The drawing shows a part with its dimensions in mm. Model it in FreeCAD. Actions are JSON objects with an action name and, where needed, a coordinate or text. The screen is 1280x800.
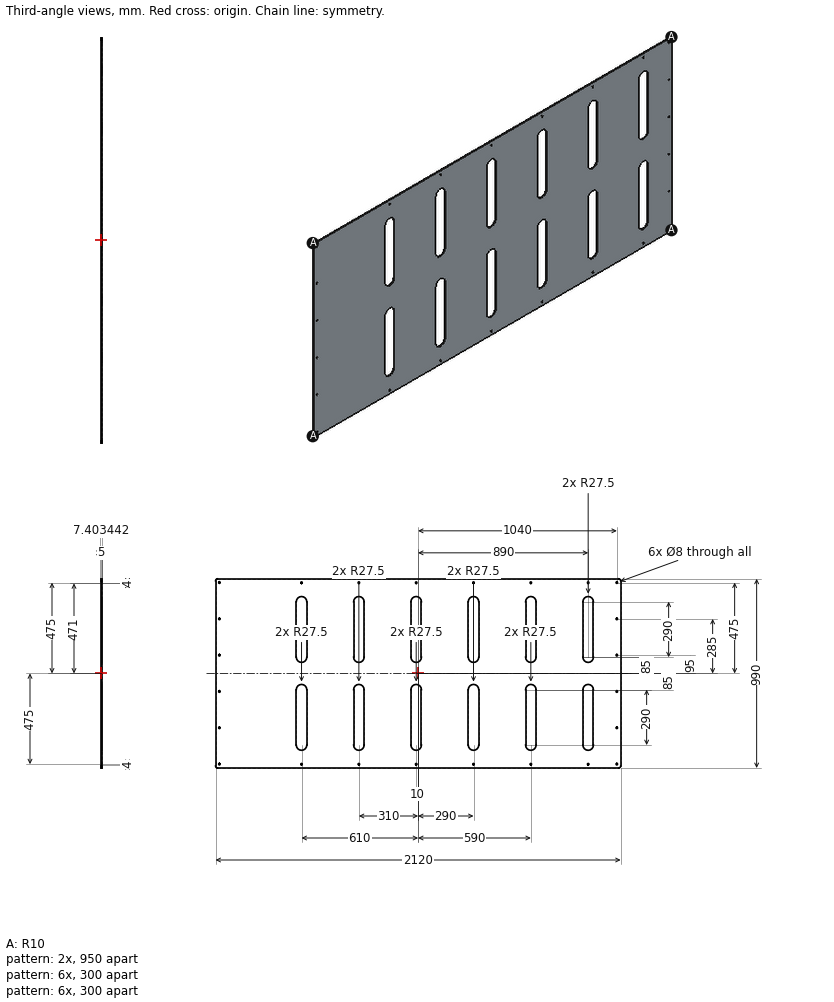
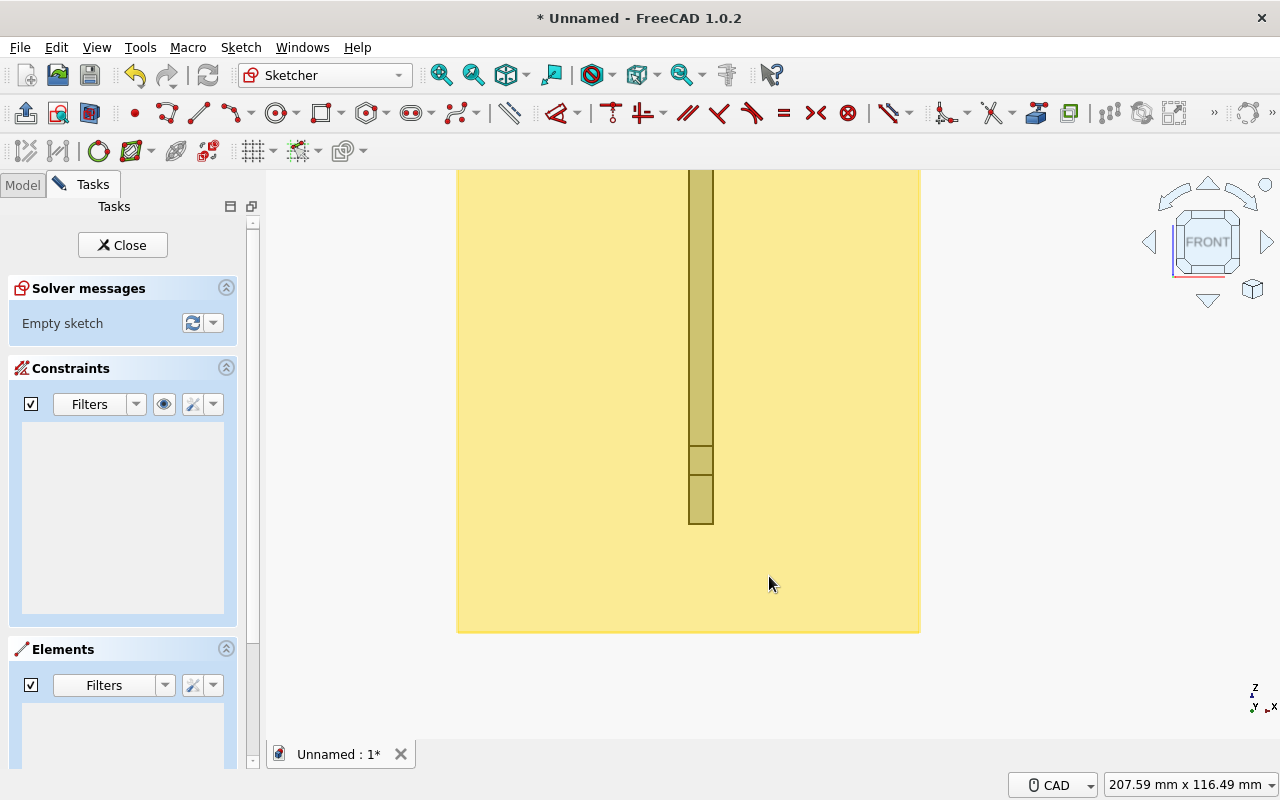
{"action": "scroll", "coordinate": [686, 434], "scroll_direction": "up", "scroll_amount": 12}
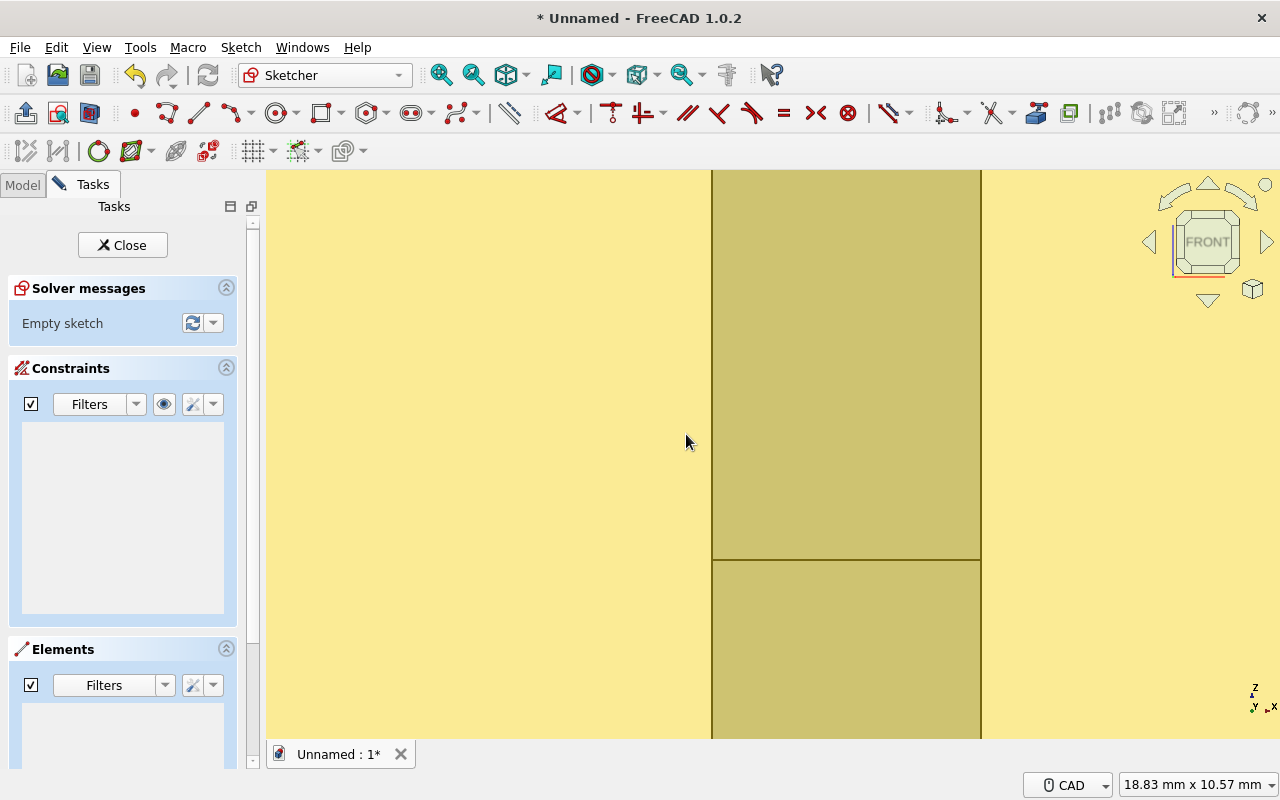
{"action": "key", "text": "g m"}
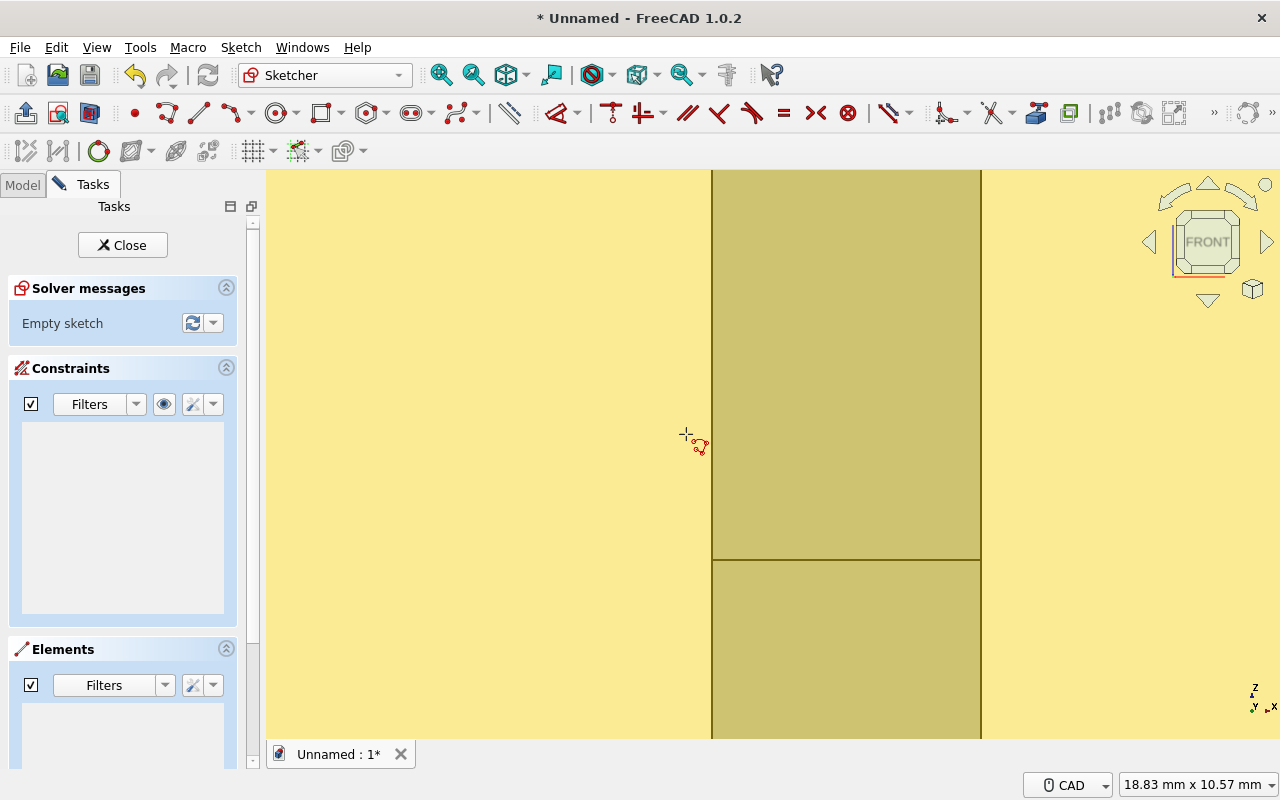
{"action": "left_click", "coordinate": [582, 345]}
{"action": "left_click", "coordinate": [981, 345]}
{"action": "left_click", "coordinate": [981, 560]}
{"action": "left_click", "coordinate": [712, 560]}
{"action": "left_click", "coordinate": [582, 346]}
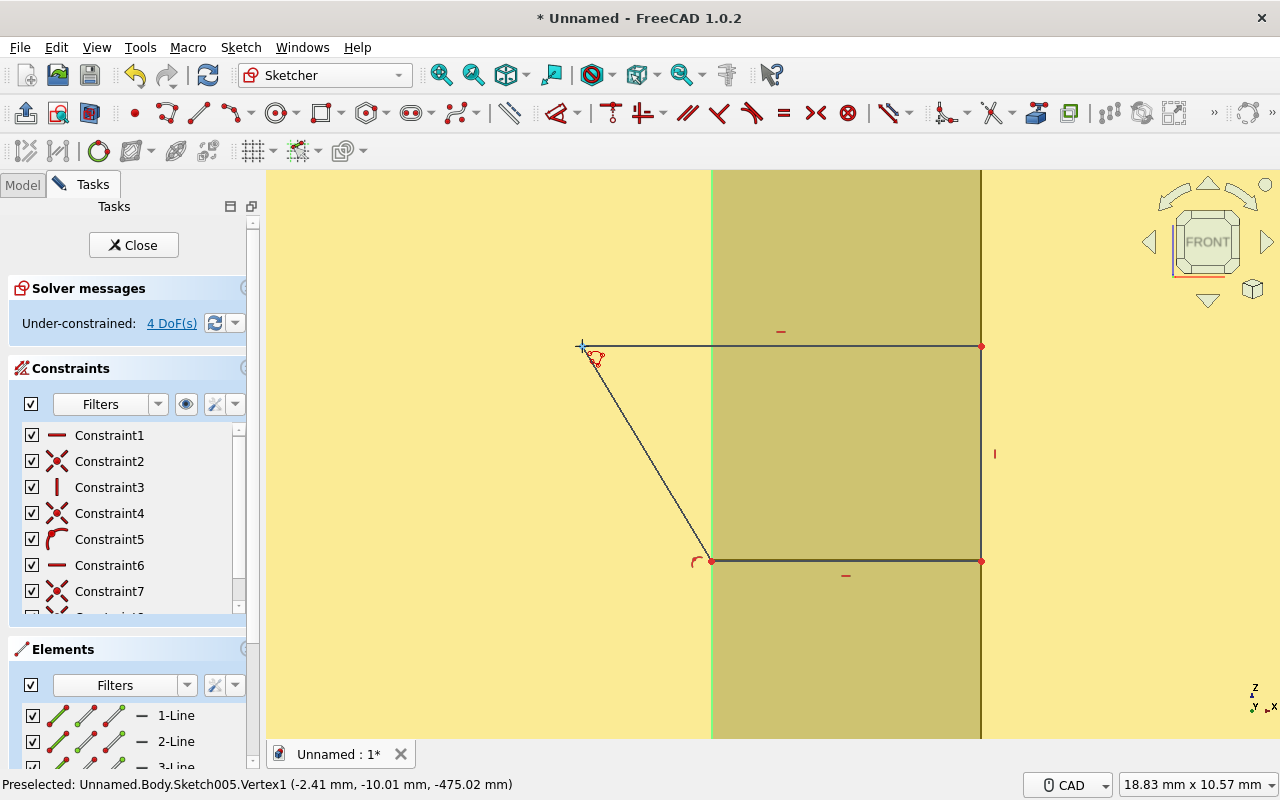
{"action": "left_click", "coordinate": [200, 114]}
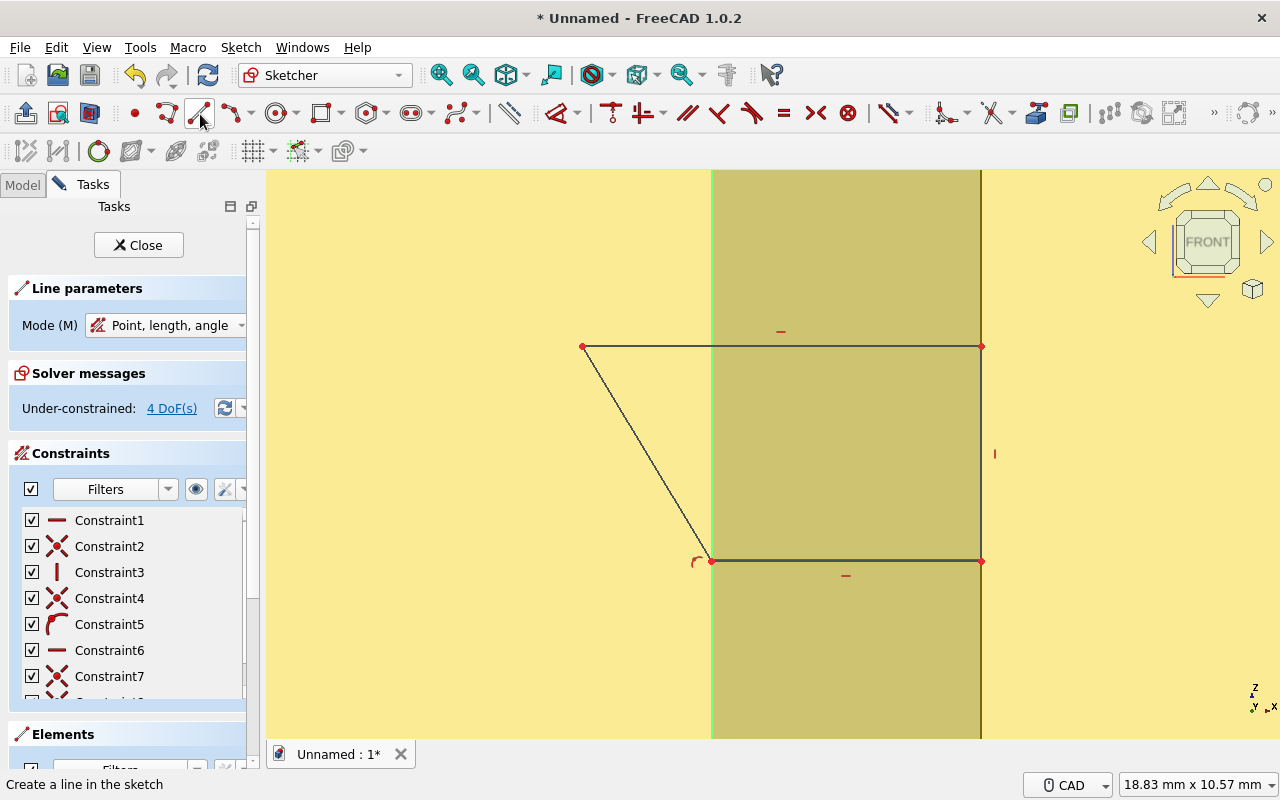
{"action": "left_click", "coordinate": [542, 345]}
{"action": "left_click", "coordinate": [423, 345]}
{"action": "key", "text": "Escape"}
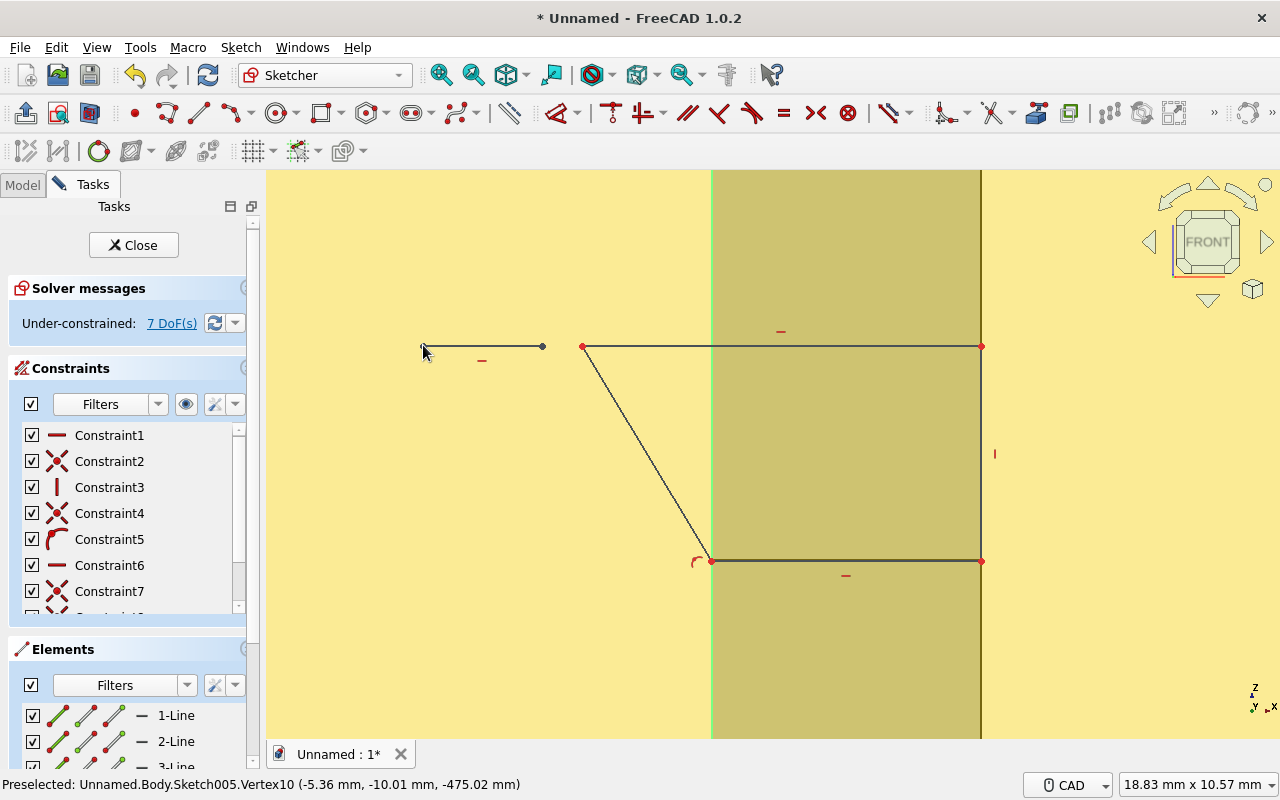
{"action": "left_click", "coordinate": [506, 346]}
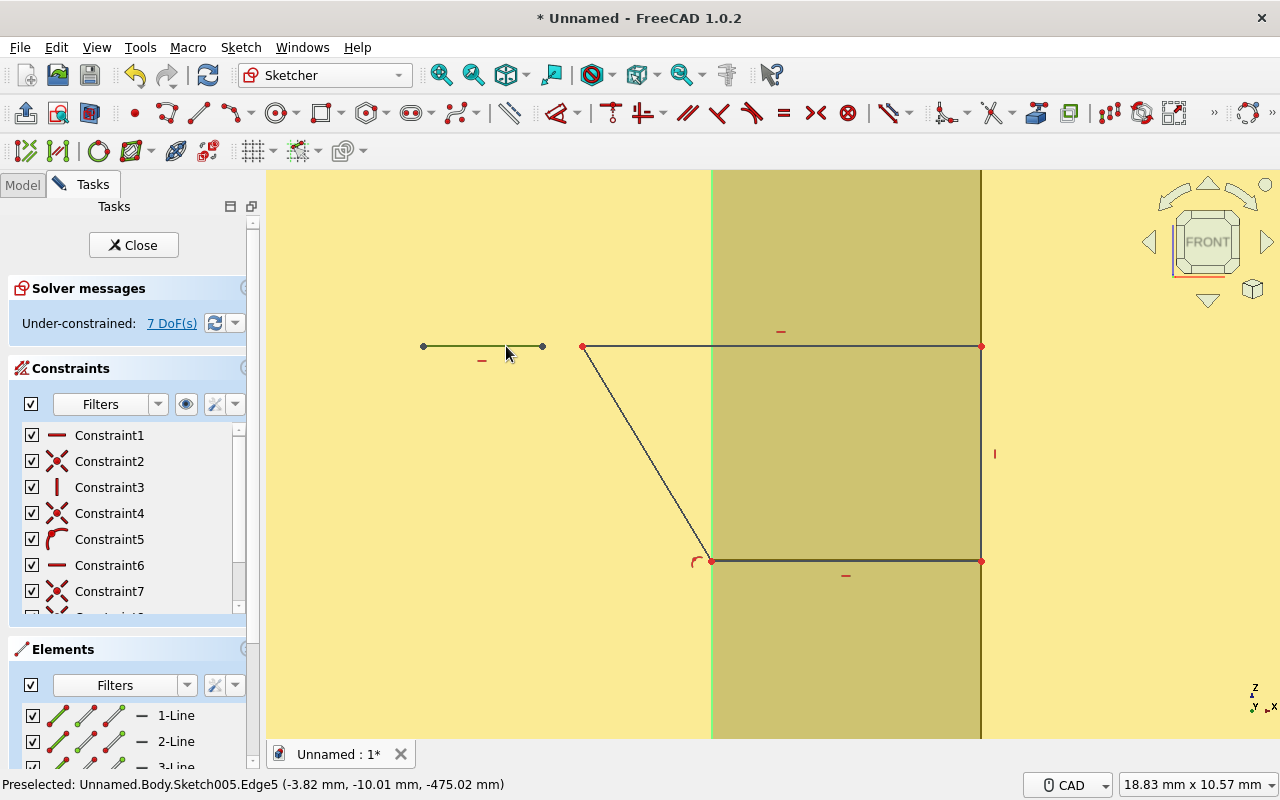
{"action": "left_click", "coordinate": [510, 114]}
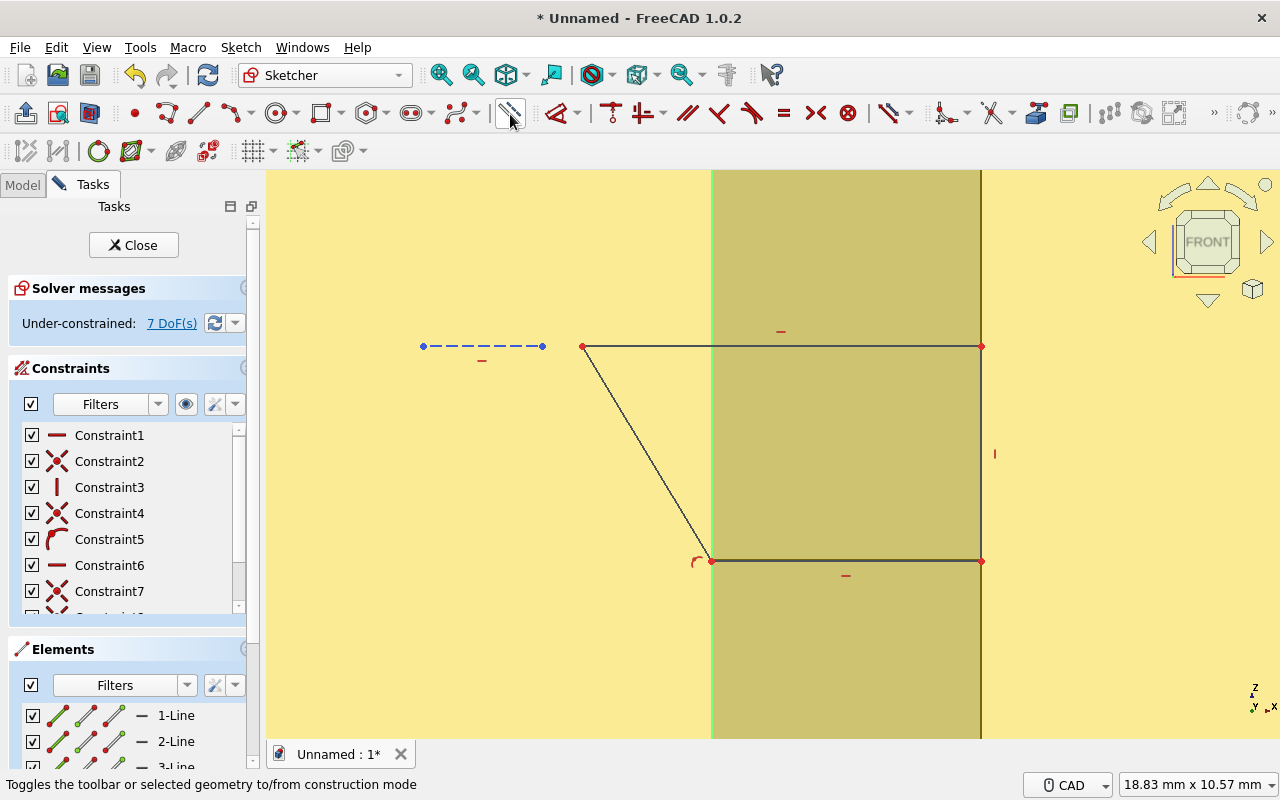
{"action": "key", "text": "d"}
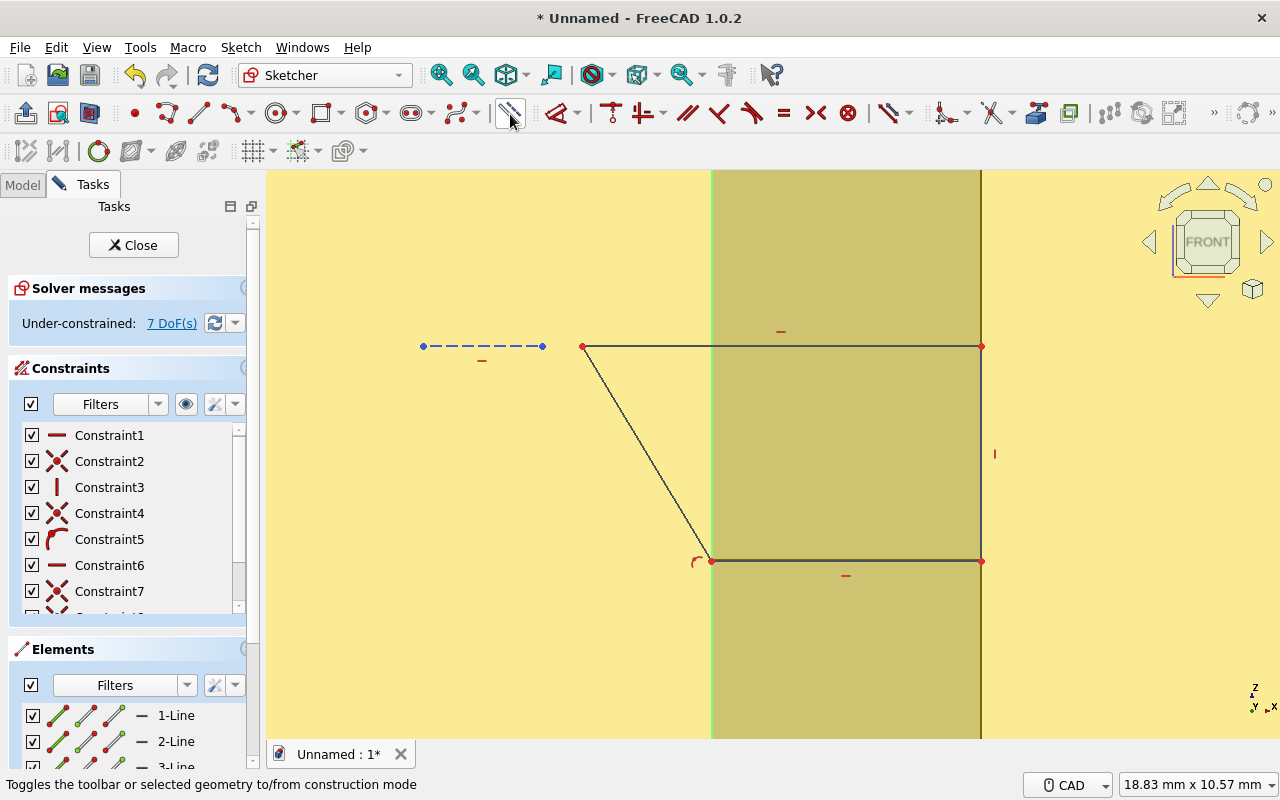
{"action": "left_click", "coordinate": [981, 411]}
{"action": "left_click", "coordinate": [1015, 454]}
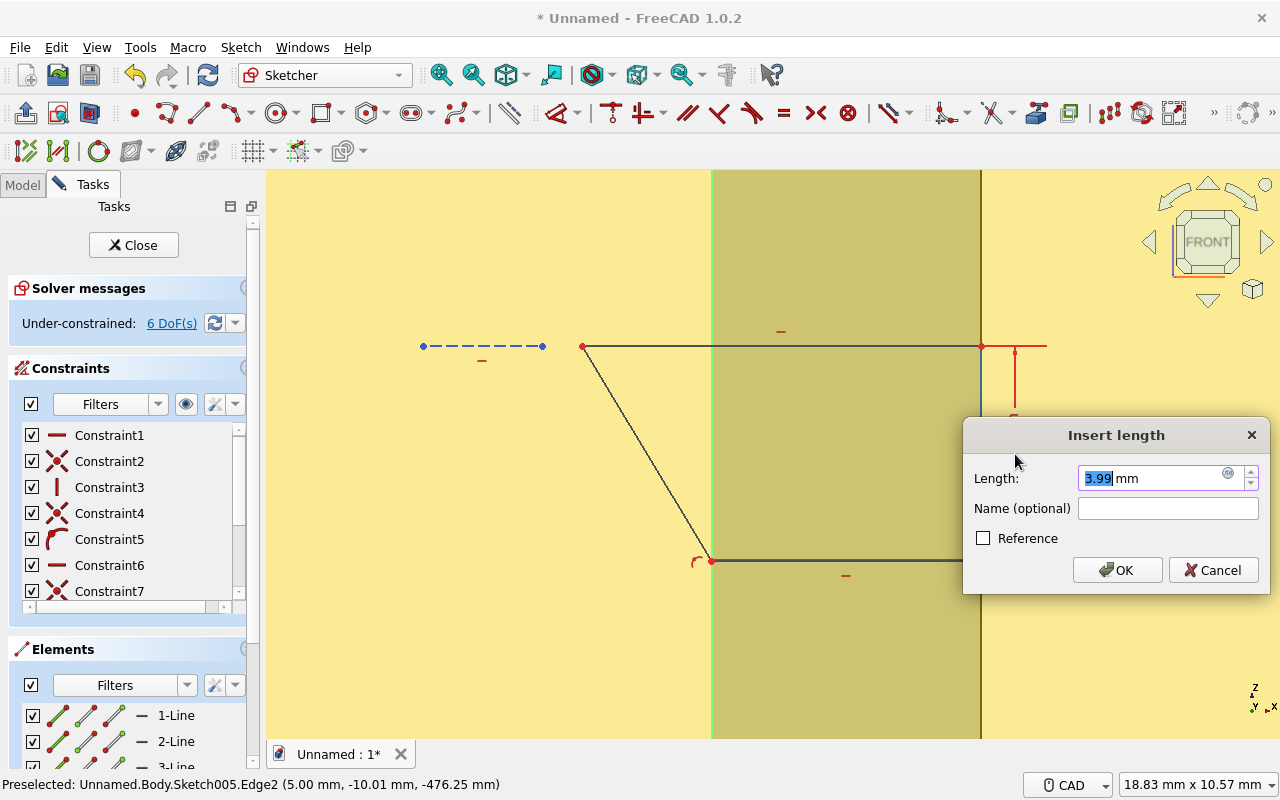
{"action": "type", "text": "4"}
{"action": "key", "text": "Return"}